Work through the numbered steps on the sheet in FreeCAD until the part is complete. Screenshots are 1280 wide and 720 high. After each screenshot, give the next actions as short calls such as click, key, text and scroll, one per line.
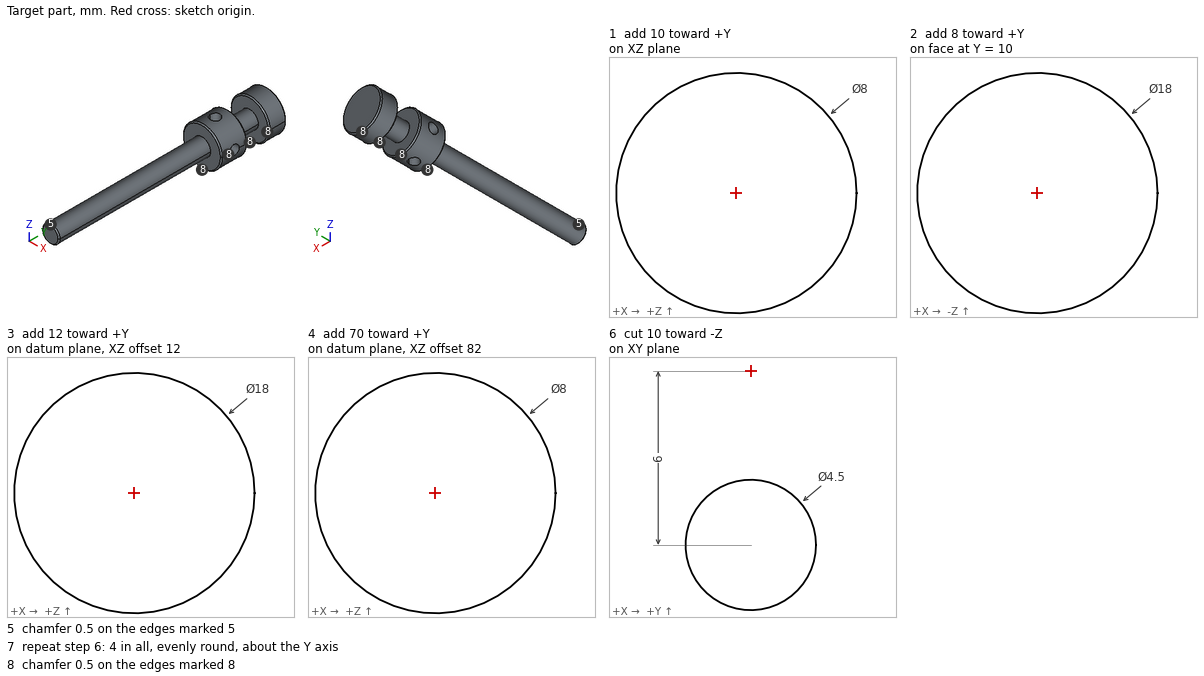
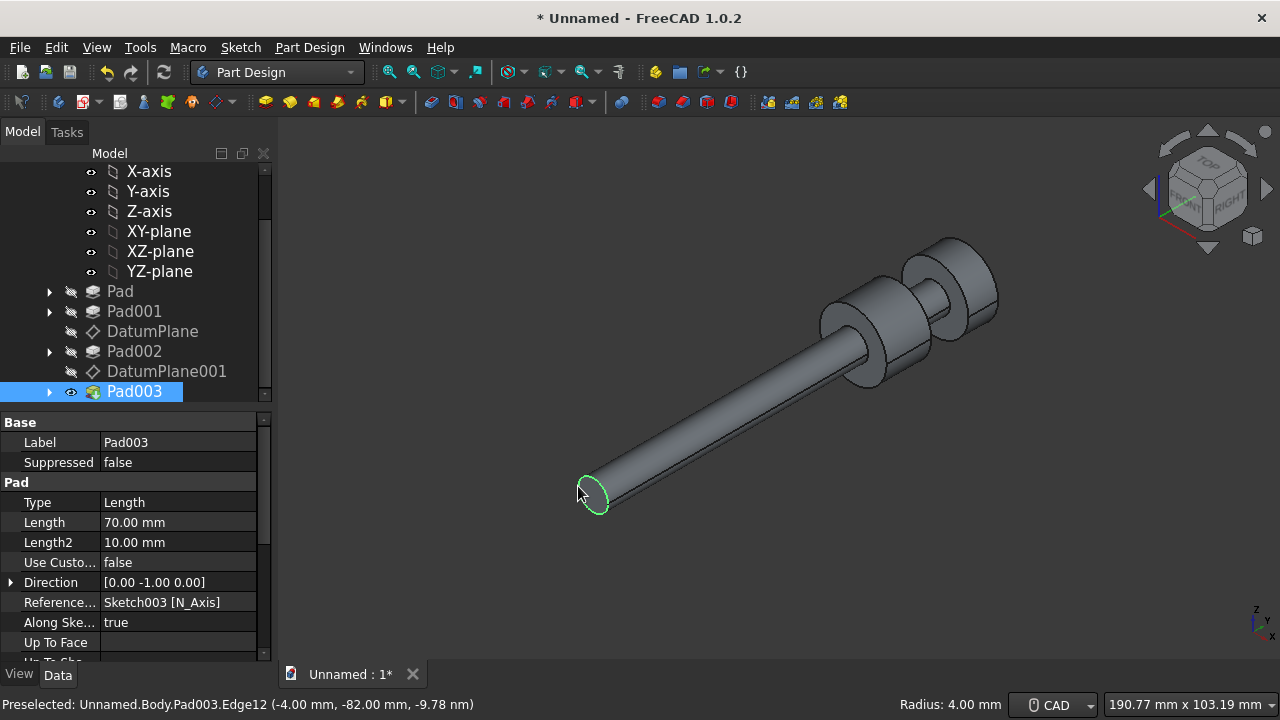
click(684, 102)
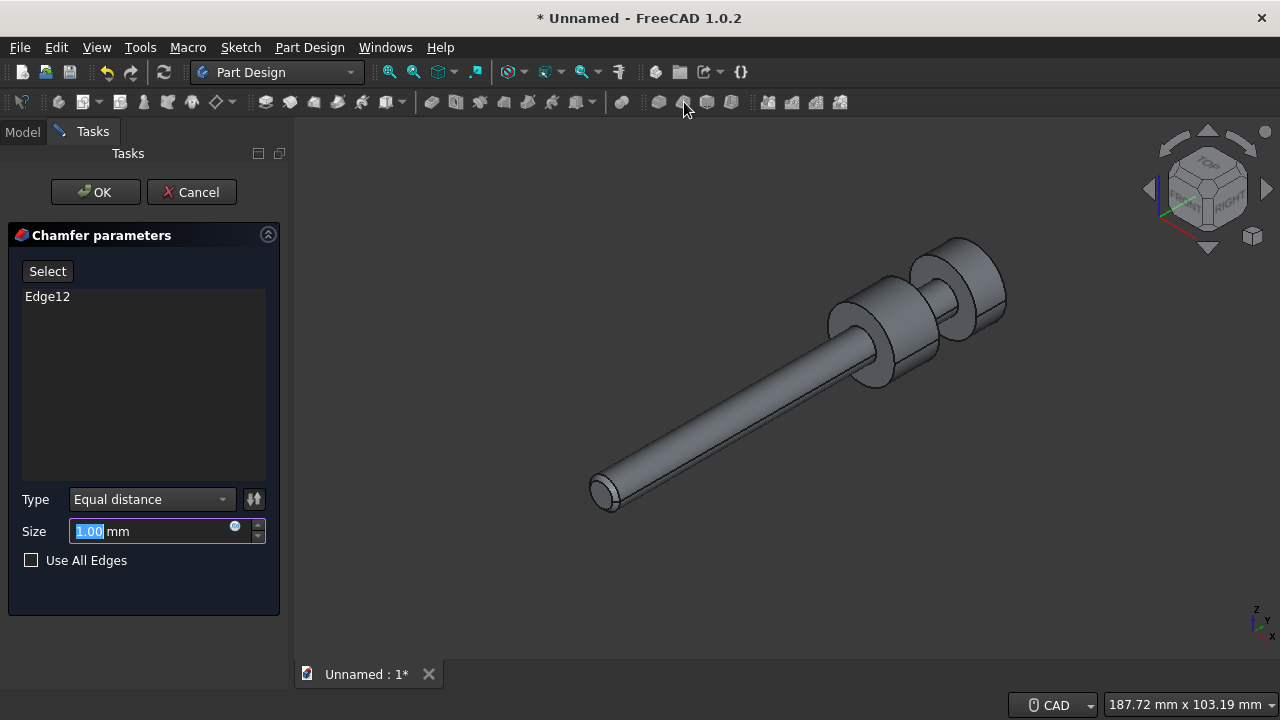
text(0.5)
key(Tab)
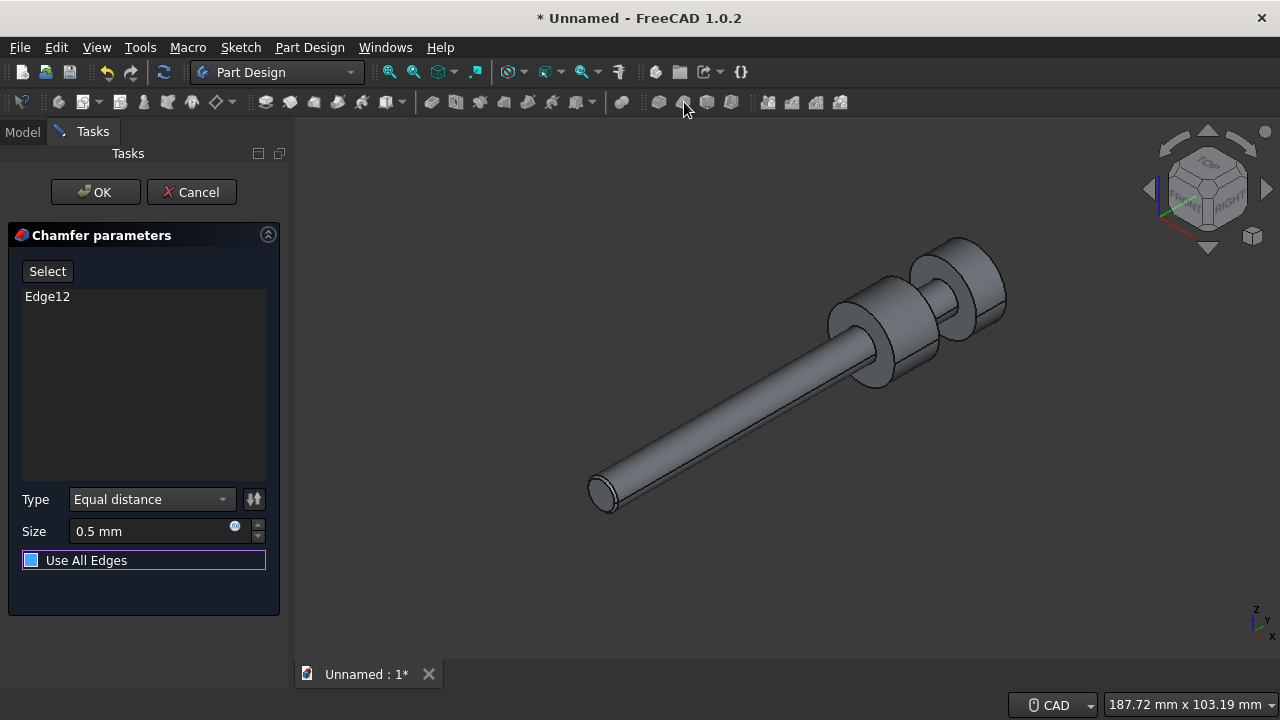
click(96, 192)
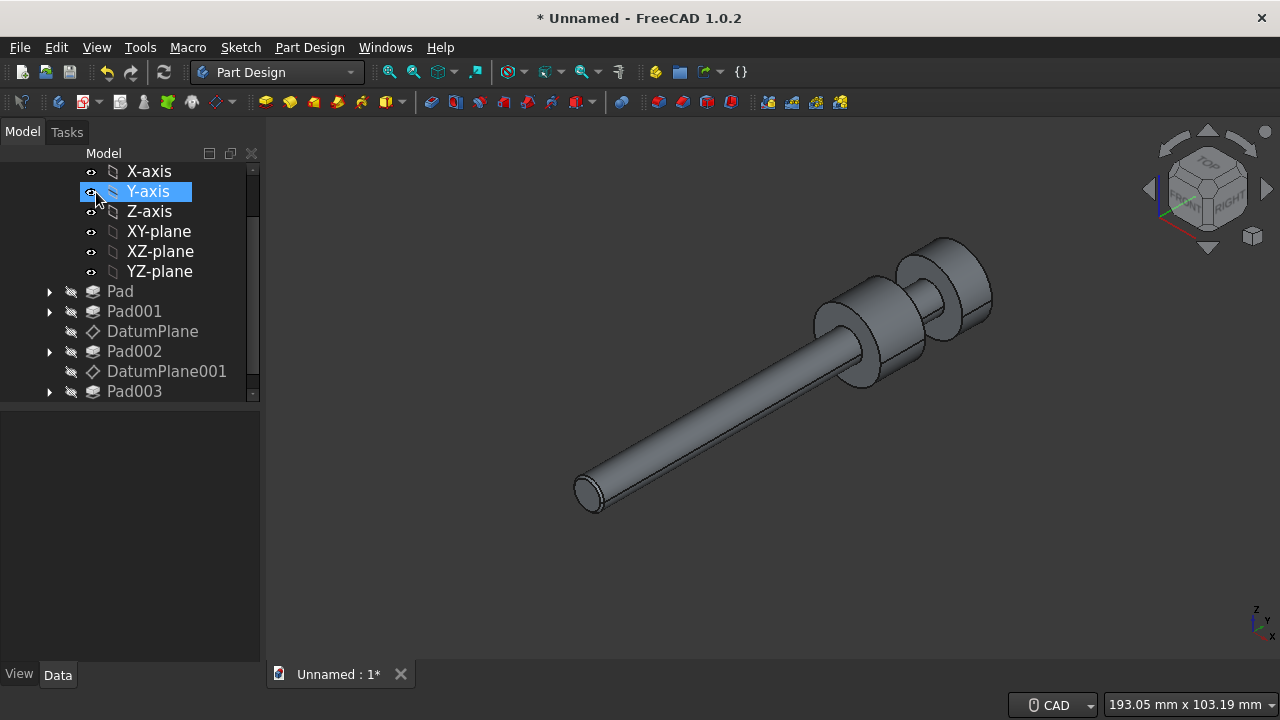
click(84, 102)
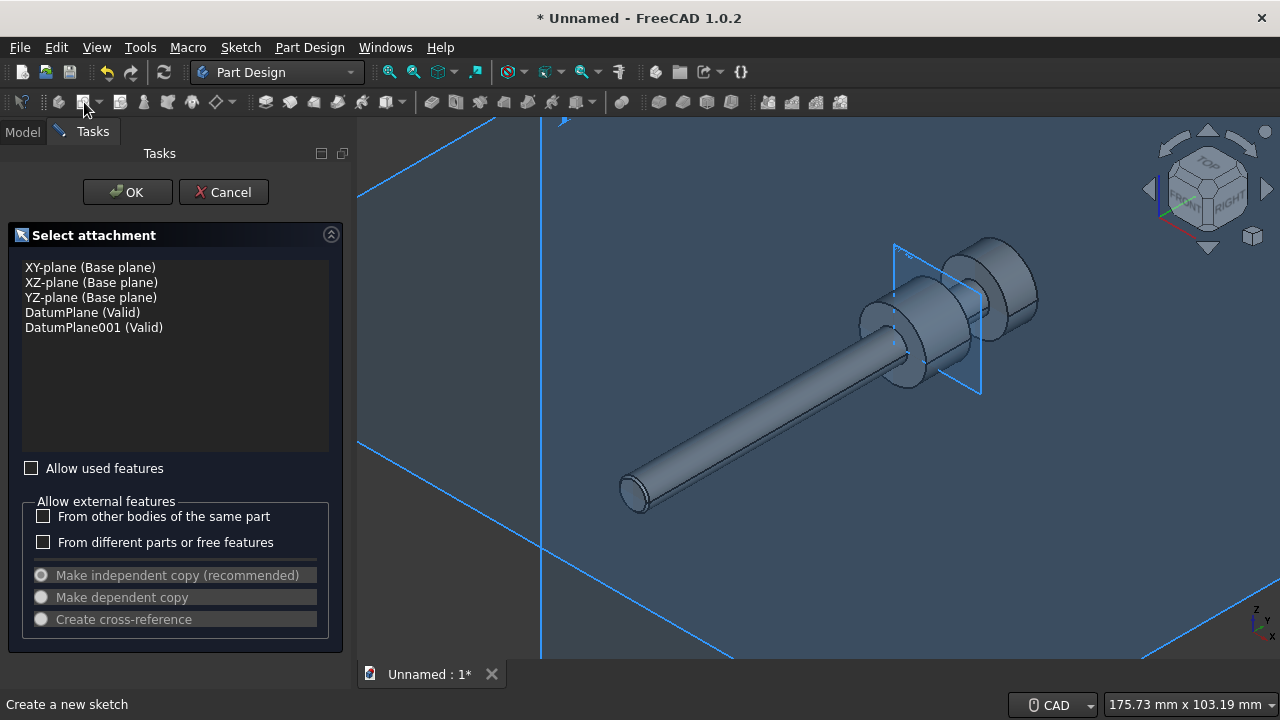
click(82, 268)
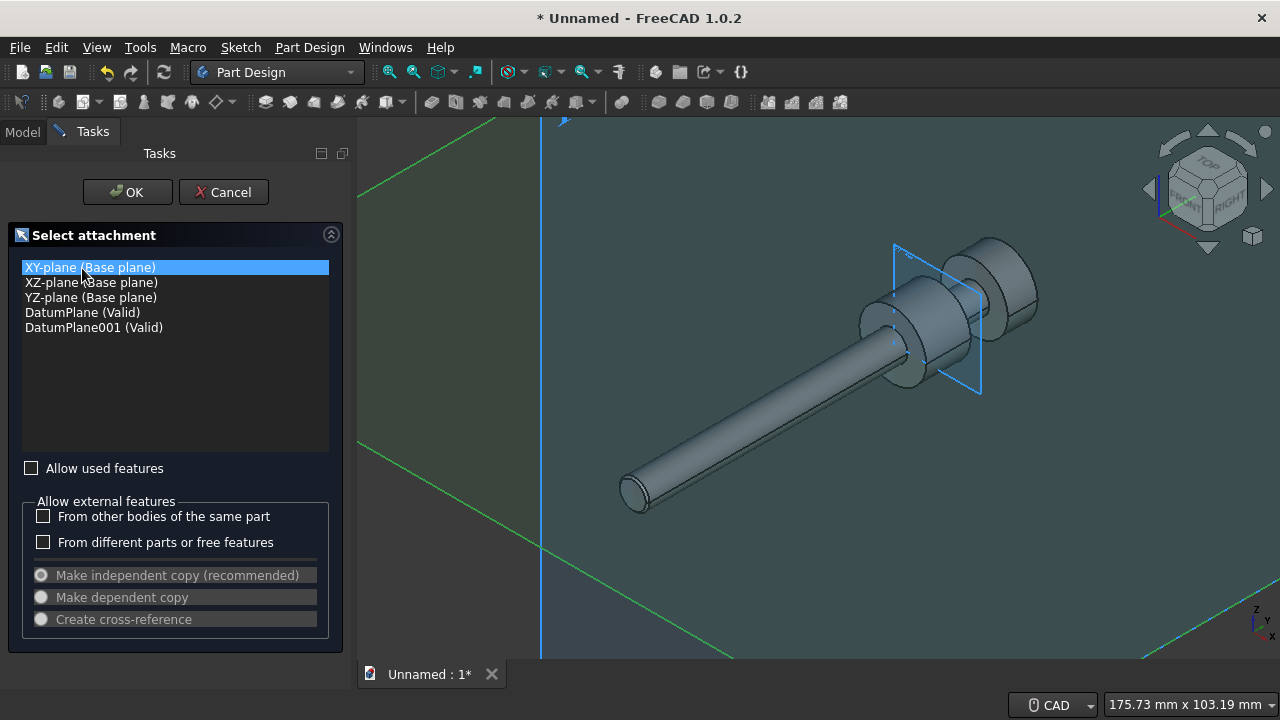
click(128, 192)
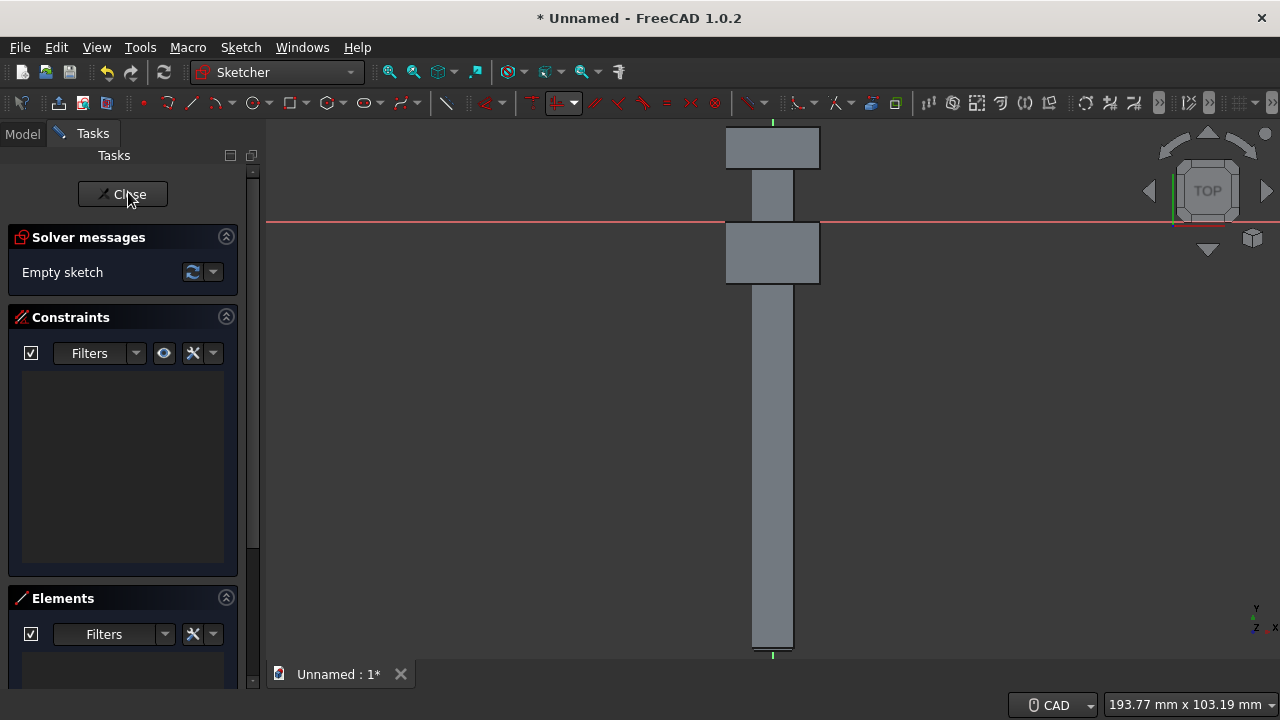
click(108, 104)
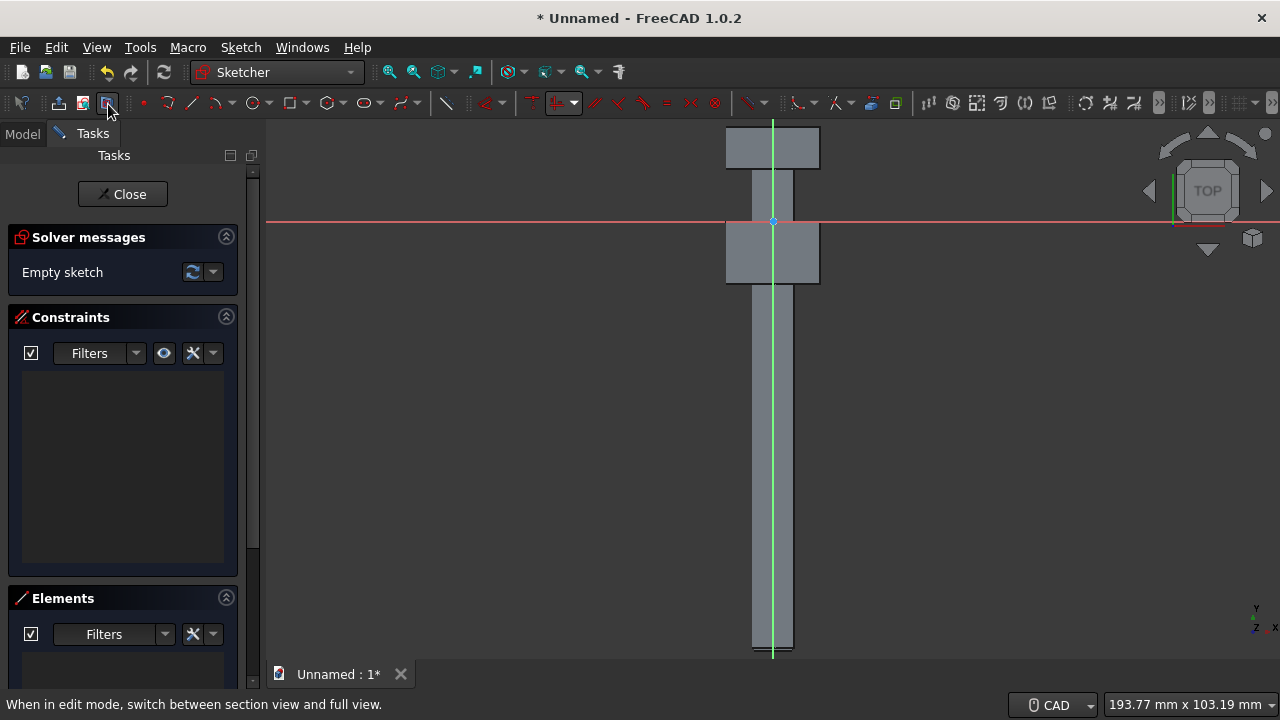
scroll(784, 220, up, 10)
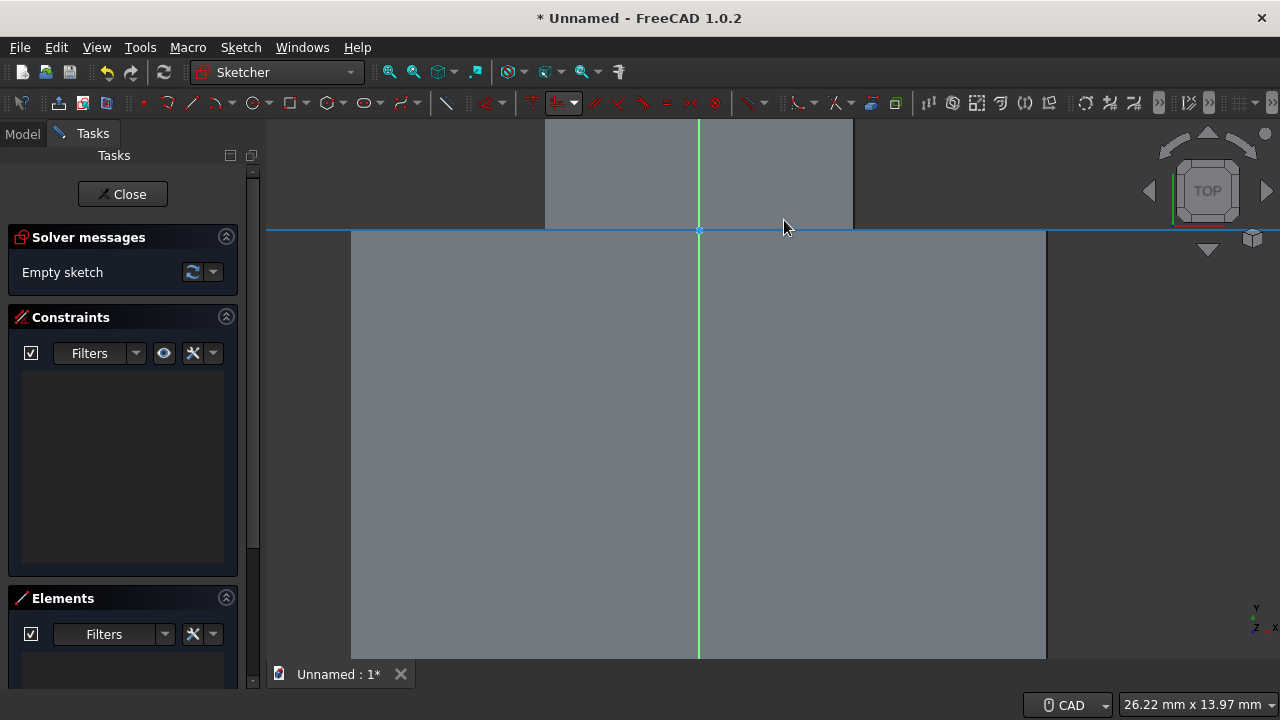
click(254, 104)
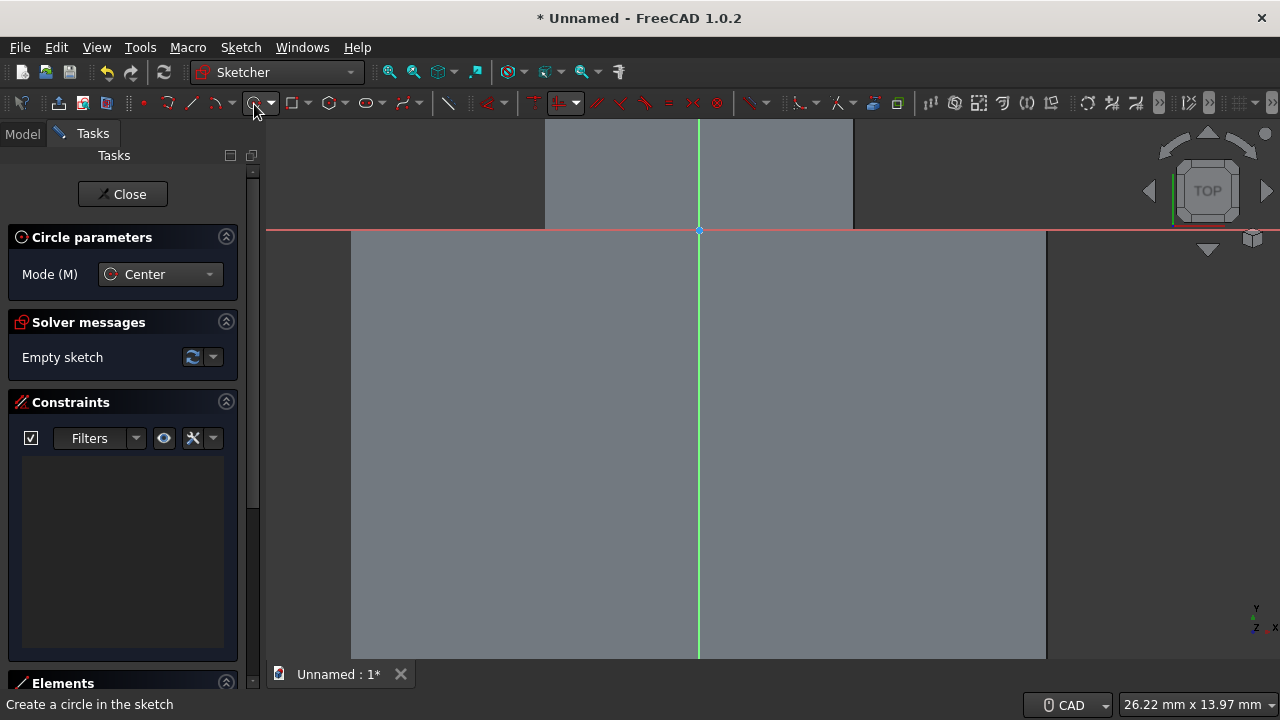
click(699, 462)
click(761, 401)
key(Escape)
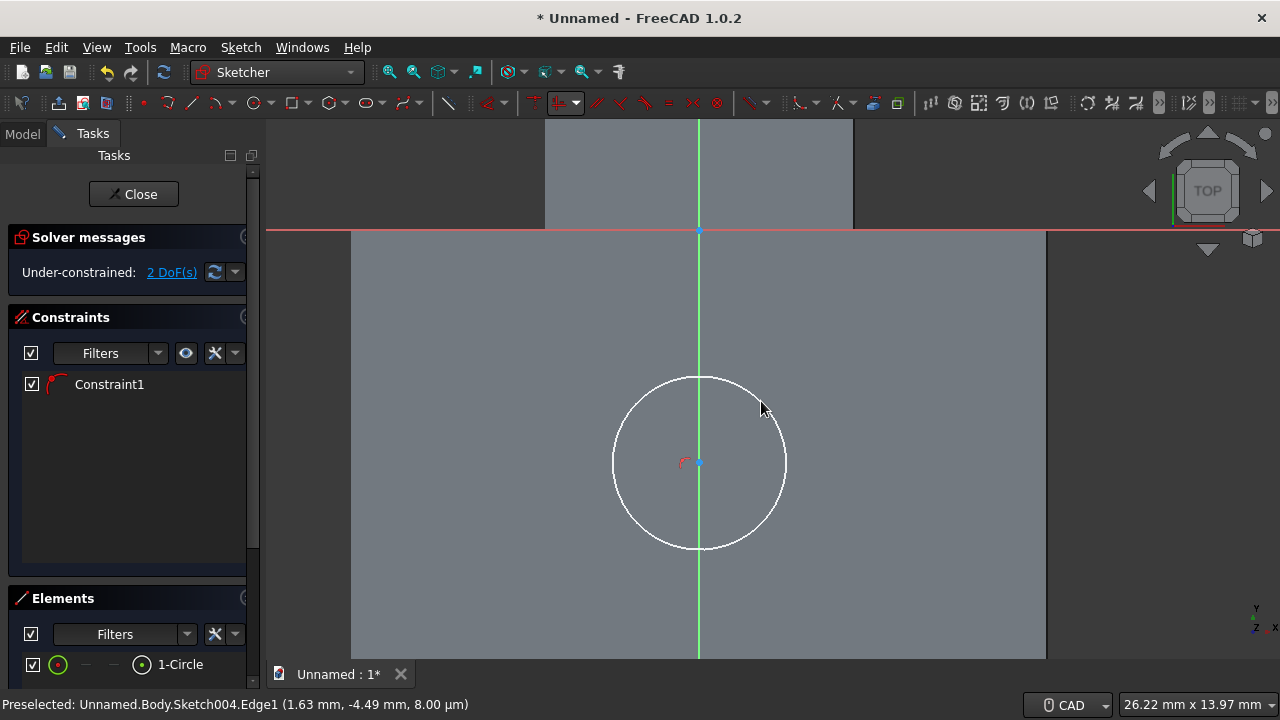
click(488, 104)